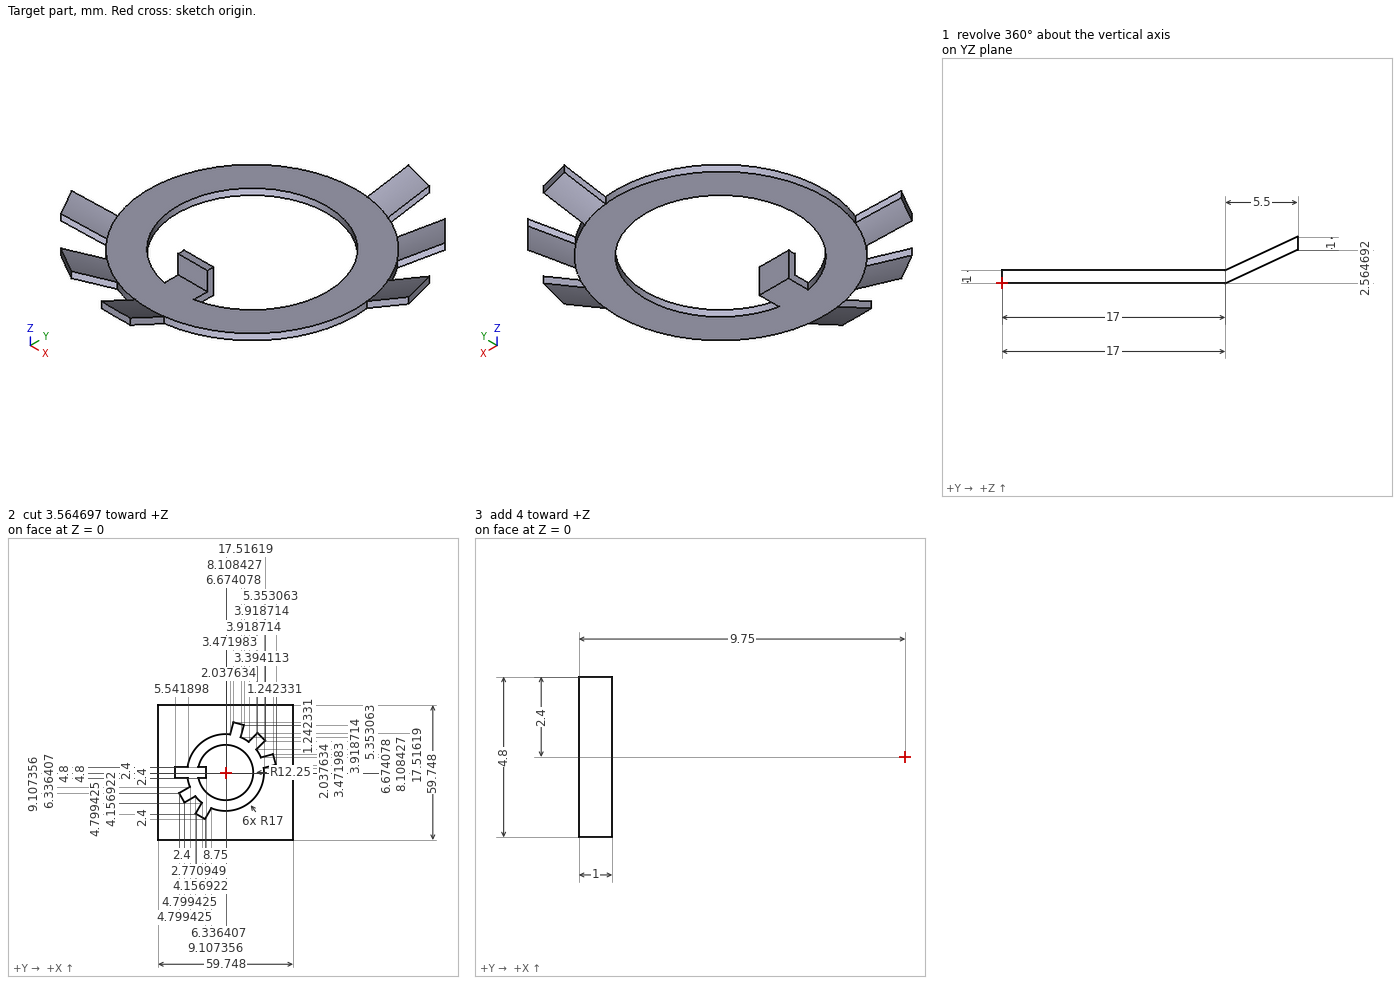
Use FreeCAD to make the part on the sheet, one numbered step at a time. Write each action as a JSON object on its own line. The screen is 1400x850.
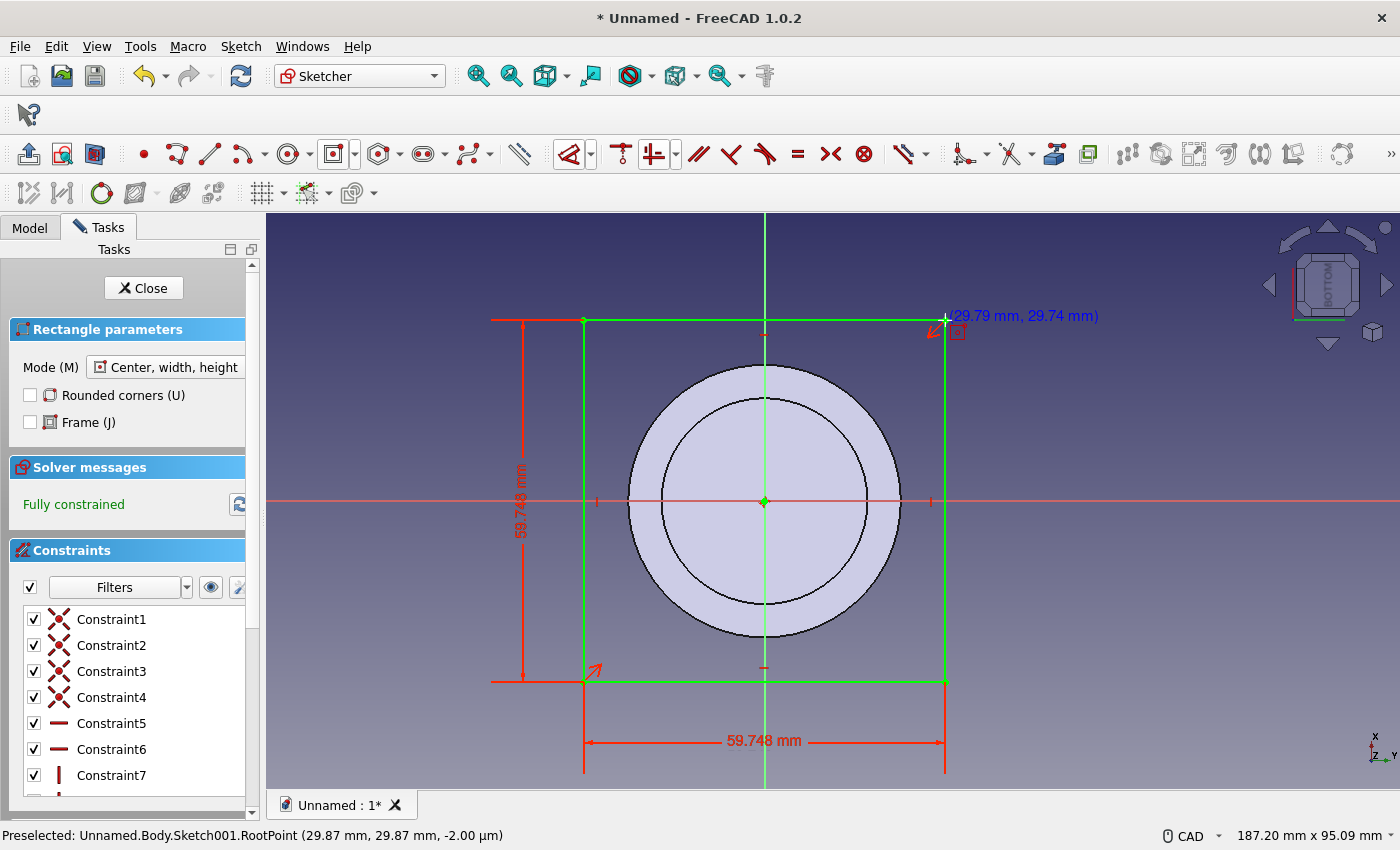
{"action": "key", "text": "g m"}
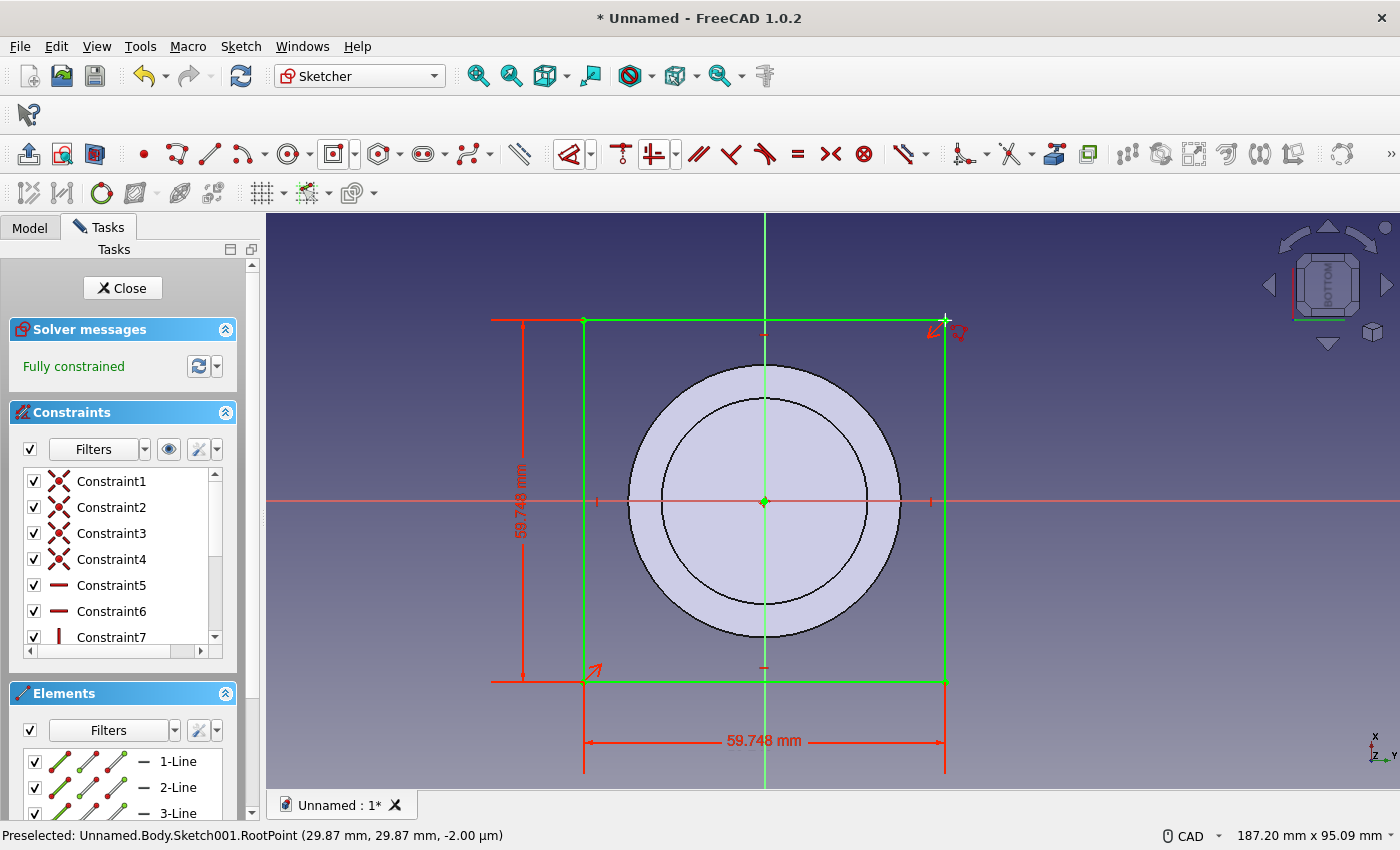
{"action": "left_click", "coordinate": [692, 516]}
{"action": "left_click", "coordinate": [712, 516]}
{"action": "left_click", "coordinate": [712, 487]}
{"action": "left_click", "coordinate": [692, 487]}
{"action": "right_click", "coordinate": [692, 487]}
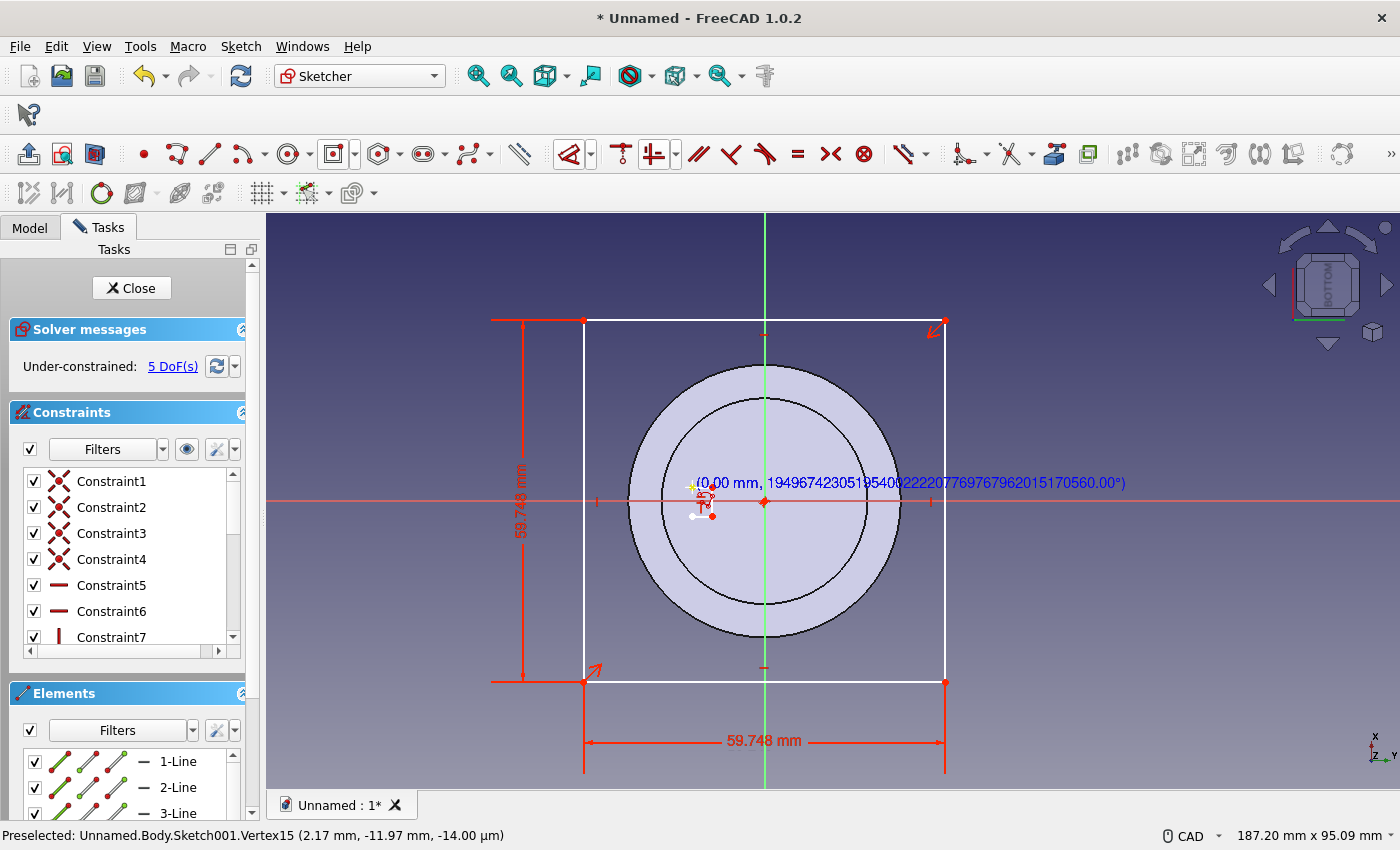
{"action": "left_click", "coordinate": [264, 154]}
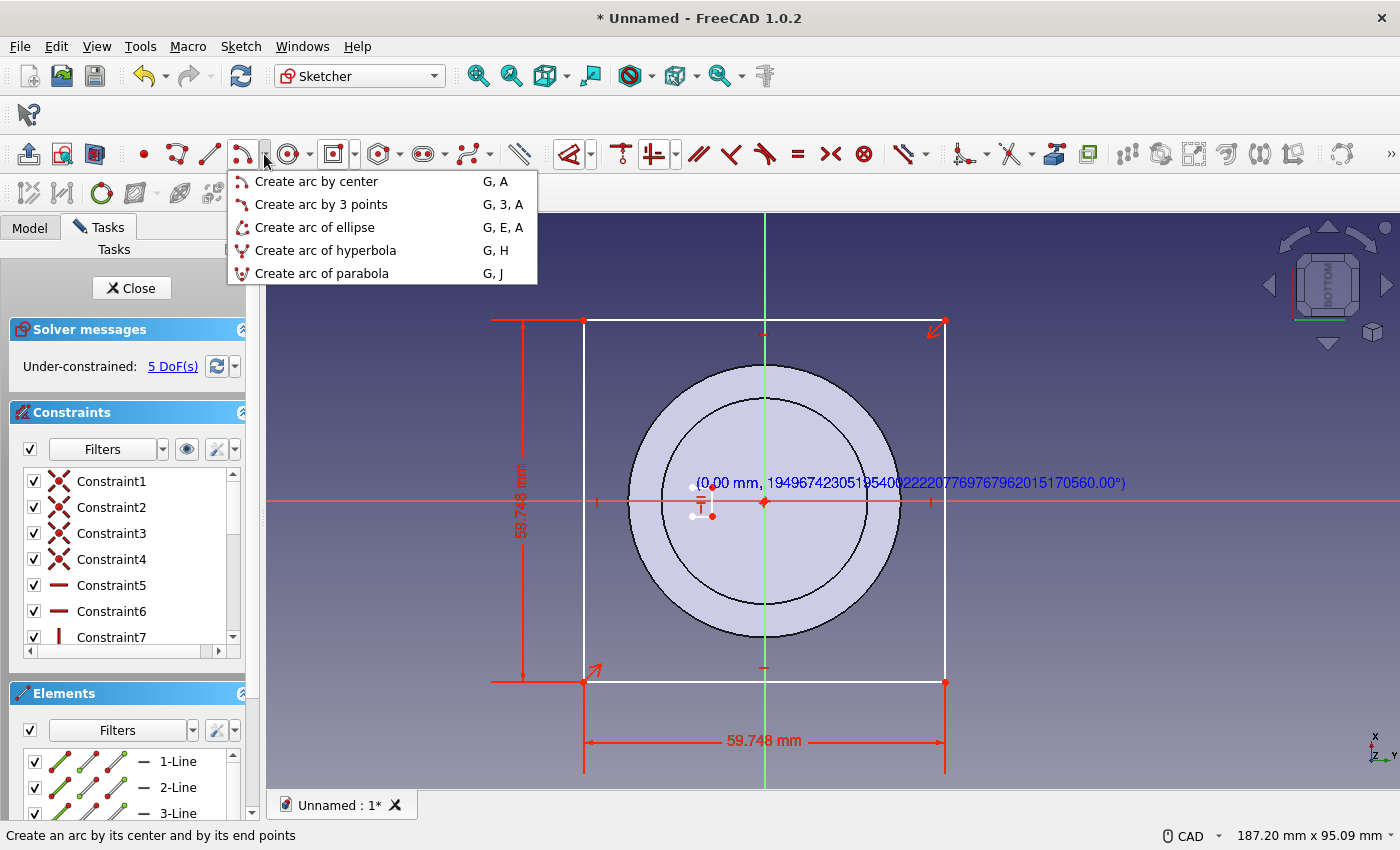
{"action": "left_click", "coordinate": [382, 204]}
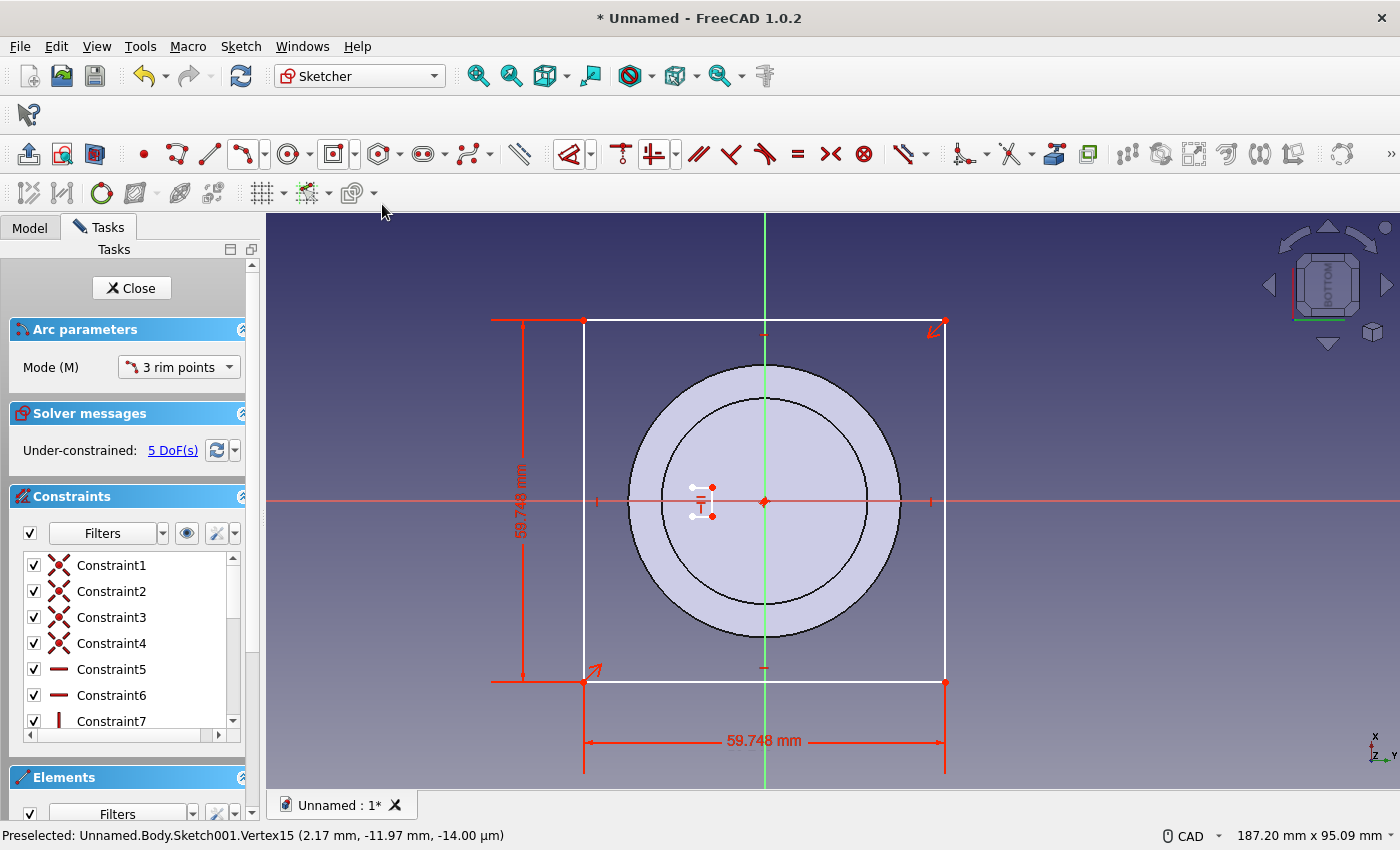
{"action": "scroll", "coordinate": [692, 487], "scroll_direction": "up", "scroll_amount": 3}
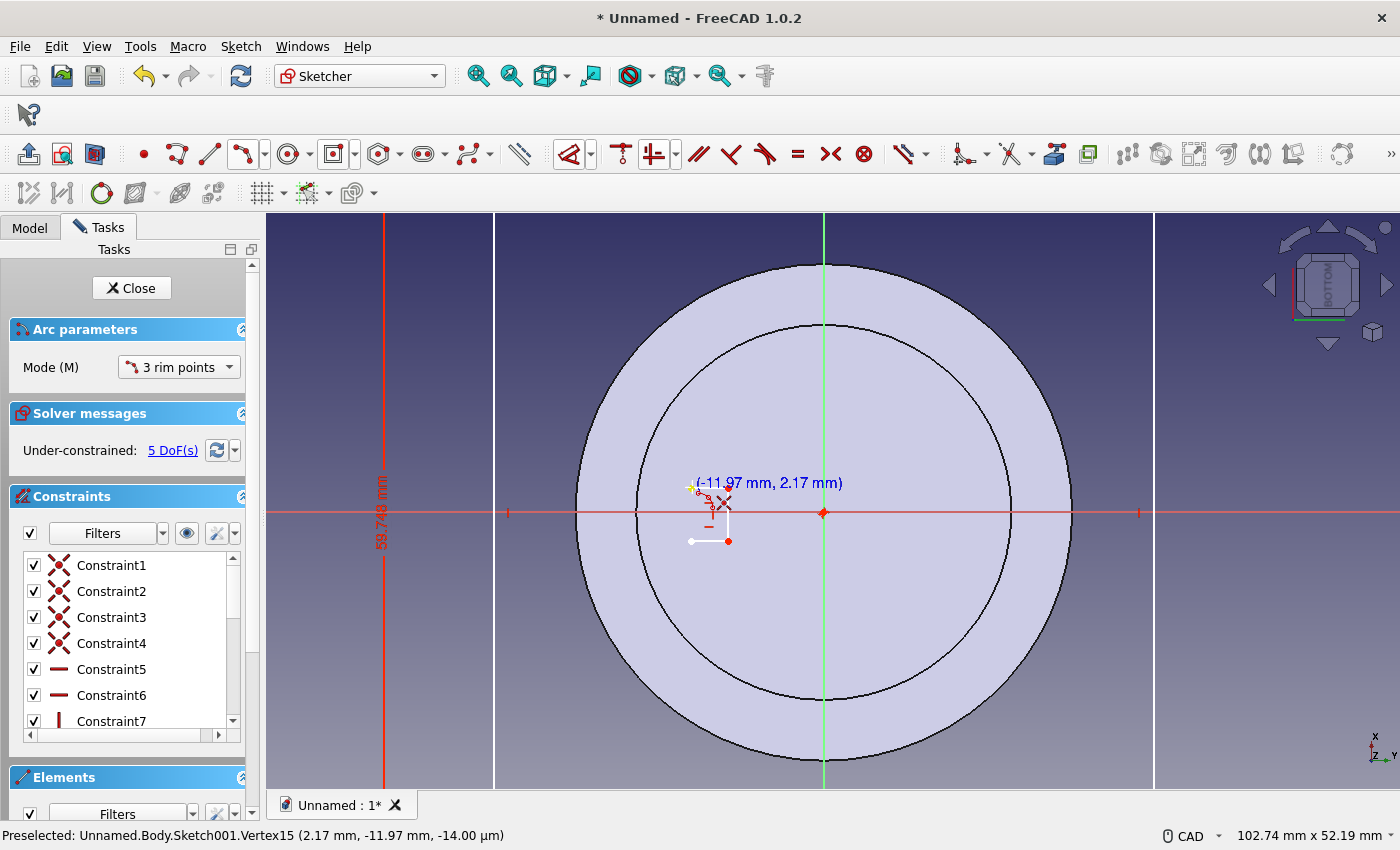
{"action": "left_click", "coordinate": [692, 488]}
{"action": "left_click", "coordinate": [692, 541]}
{"action": "left_click", "coordinate": [936, 588]}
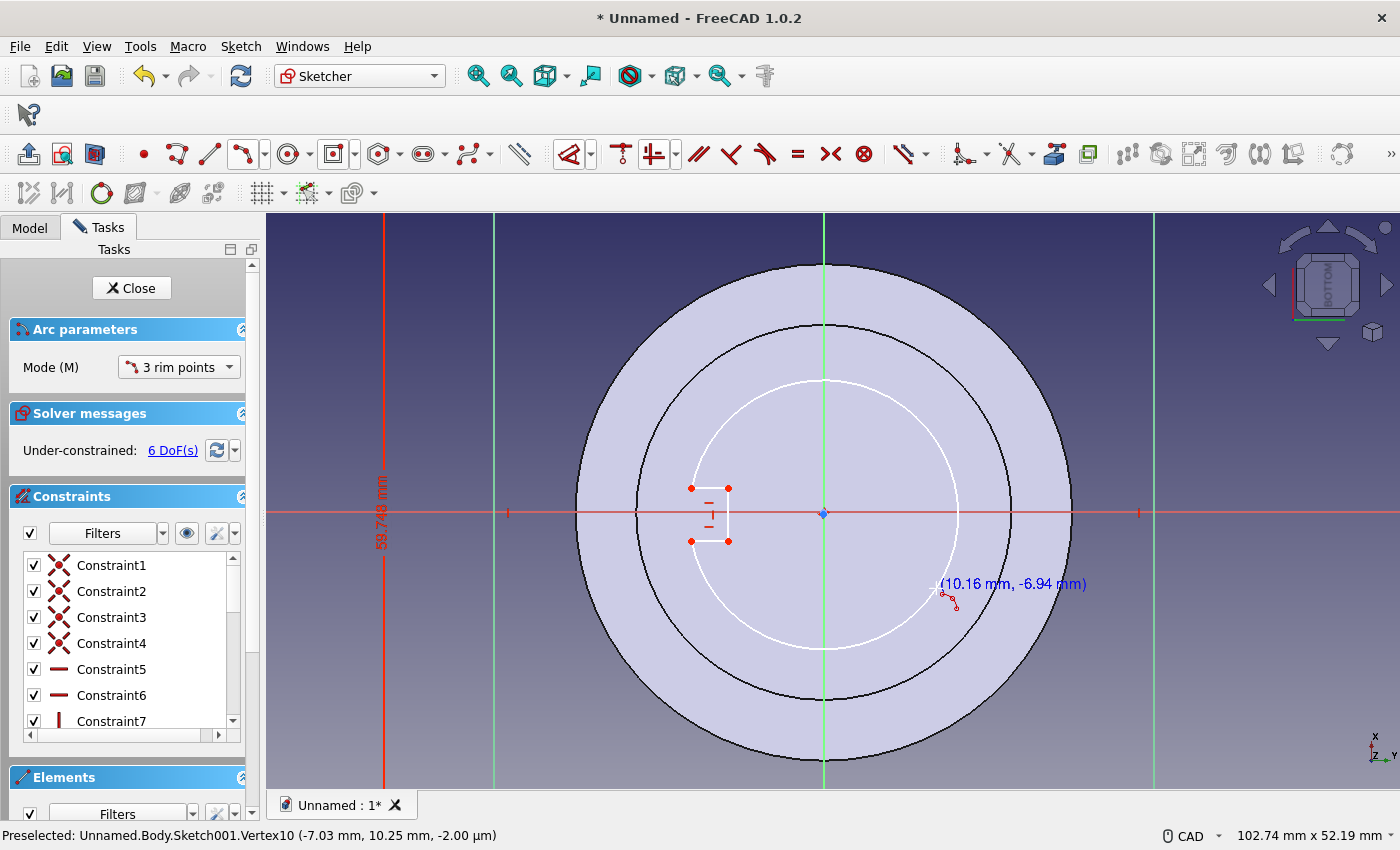
{"action": "left_click", "coordinate": [177, 154]}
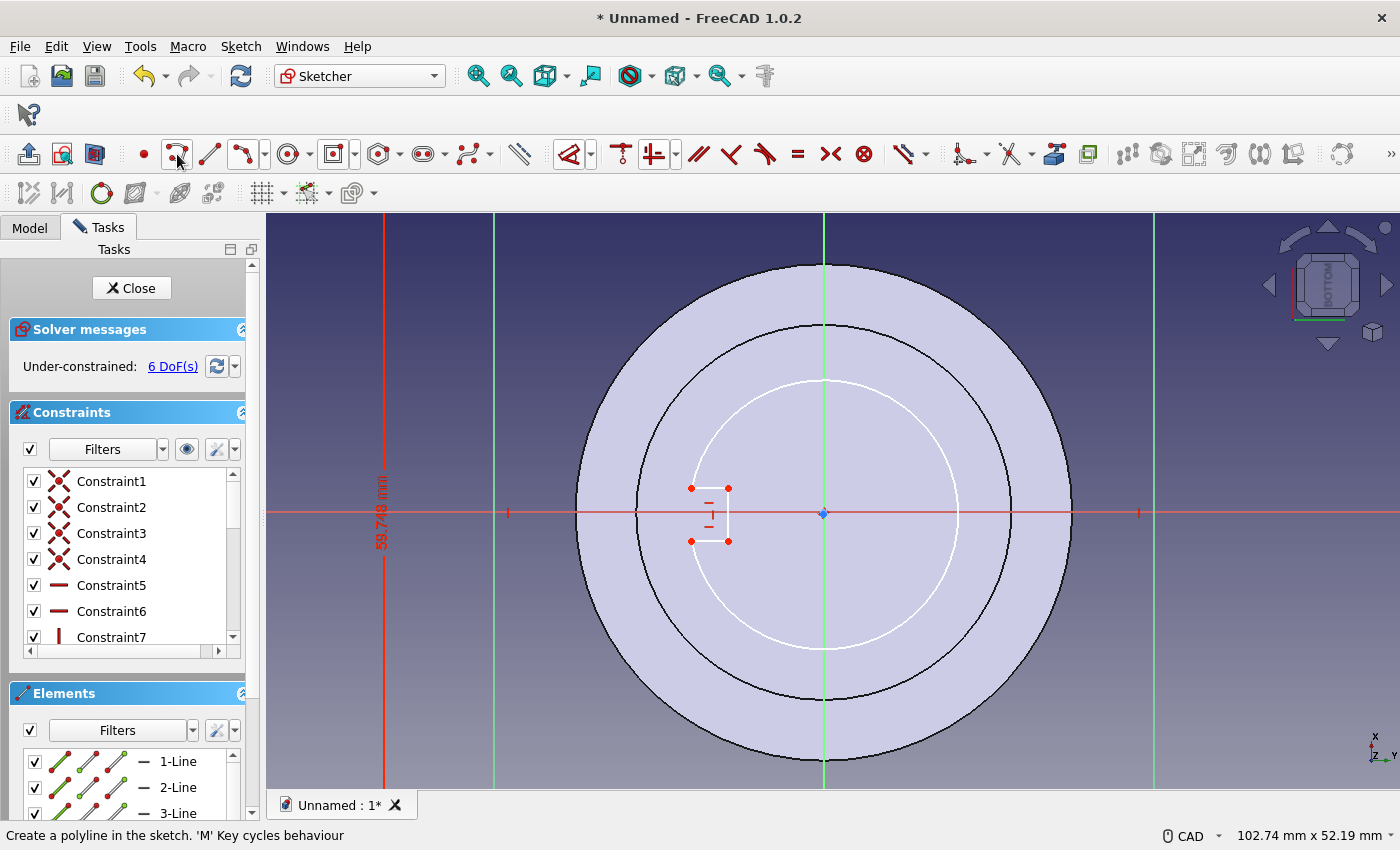
{"action": "left_click", "coordinate": [650, 582]}
{"action": "left_click", "coordinate": [597, 613]}
{"action": "left_click", "coordinate": [623, 659]}
{"action": "left_click", "coordinate": [676, 628]}
{"action": "right_click", "coordinate": [676, 628]}